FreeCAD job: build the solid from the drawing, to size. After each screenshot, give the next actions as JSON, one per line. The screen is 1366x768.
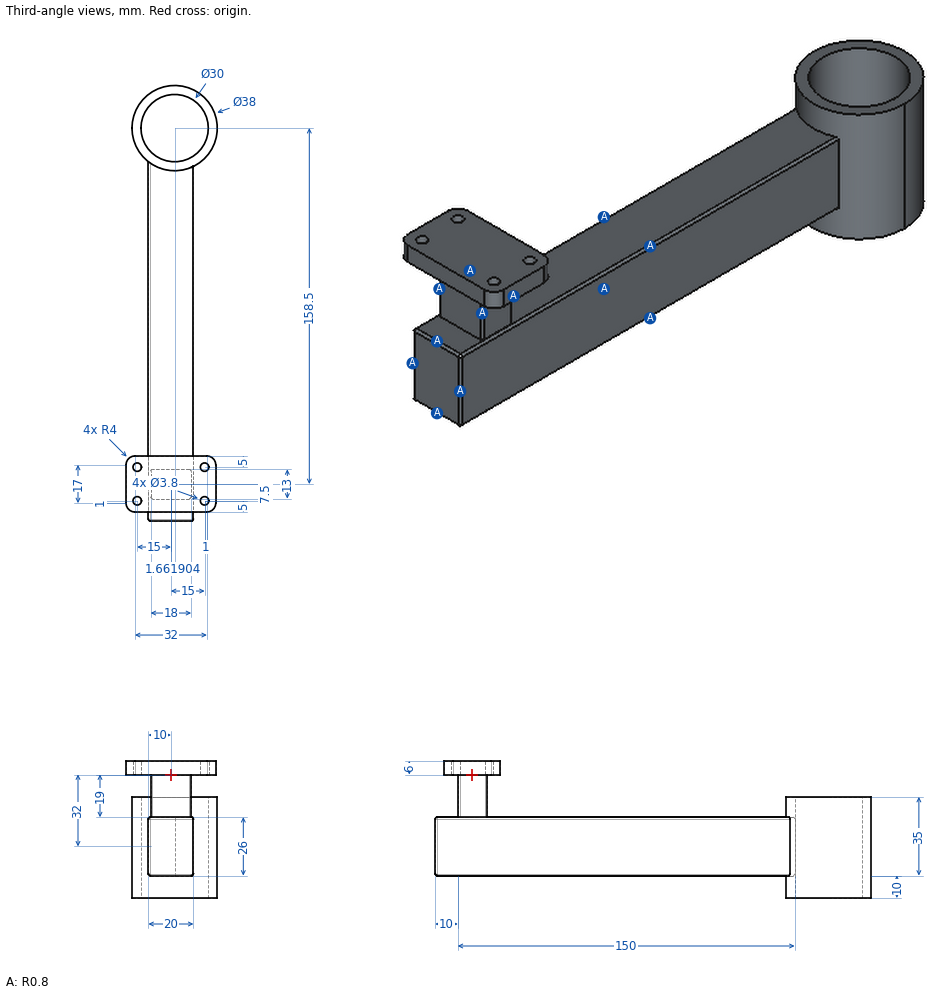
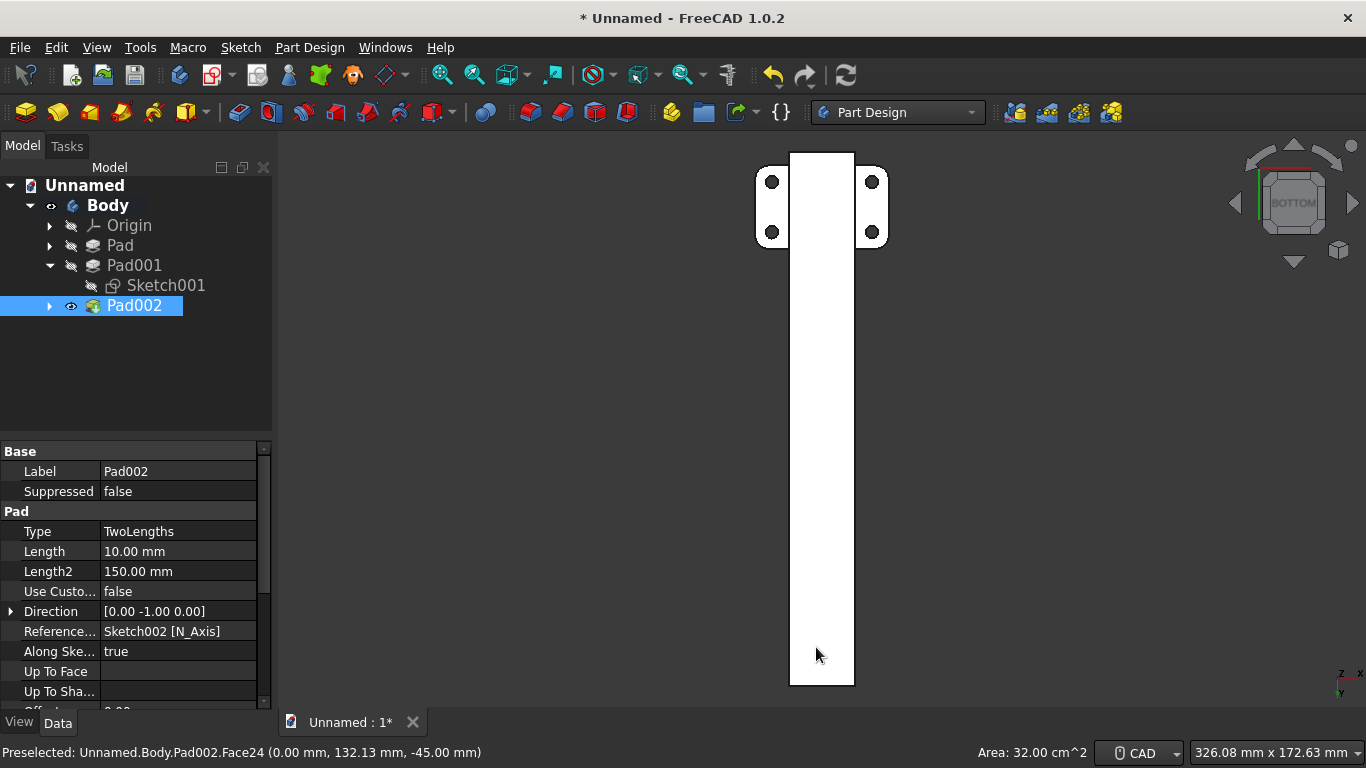
{"action": "left_click", "coordinate": [212, 76]}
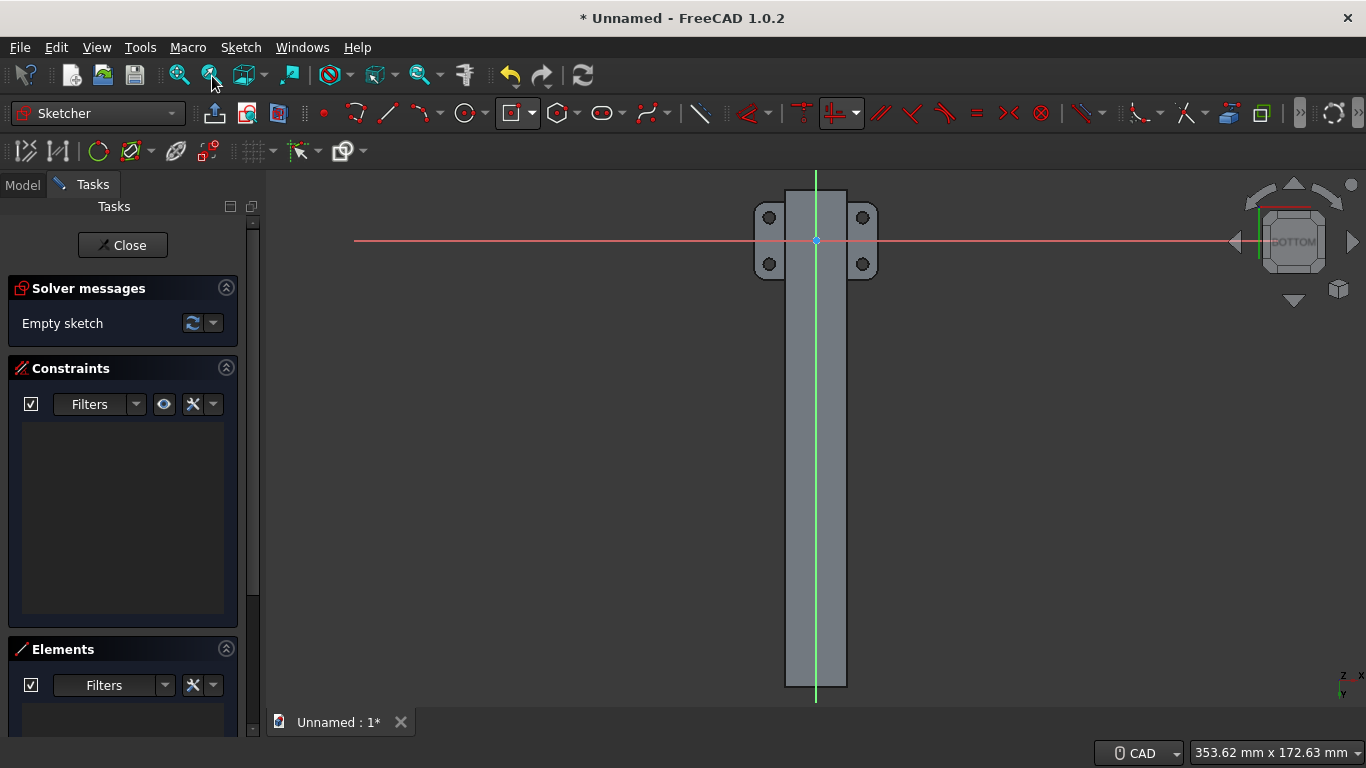
{"action": "scroll", "coordinate": [748, 438], "scroll_direction": "down", "scroll_amount": 5}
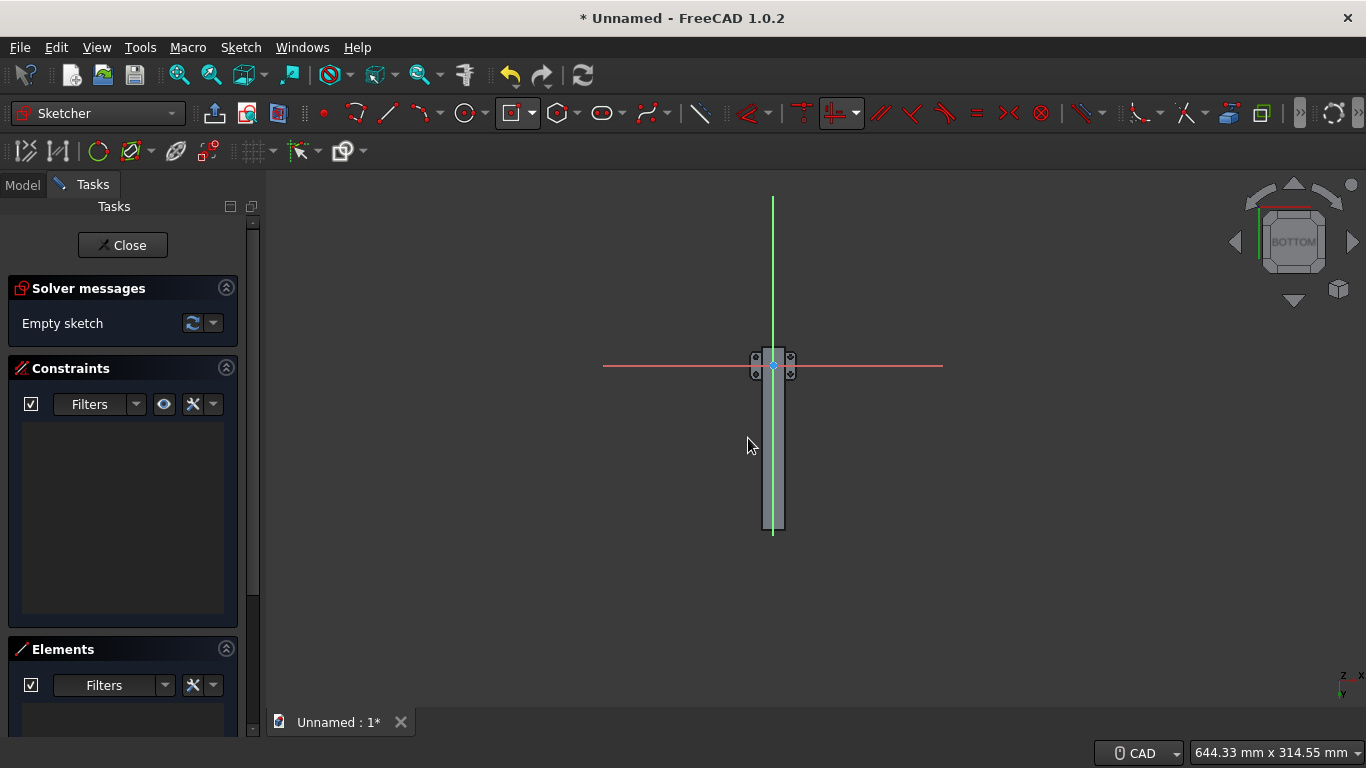
{"action": "scroll", "coordinate": [780, 564], "scroll_direction": "up", "scroll_amount": 10}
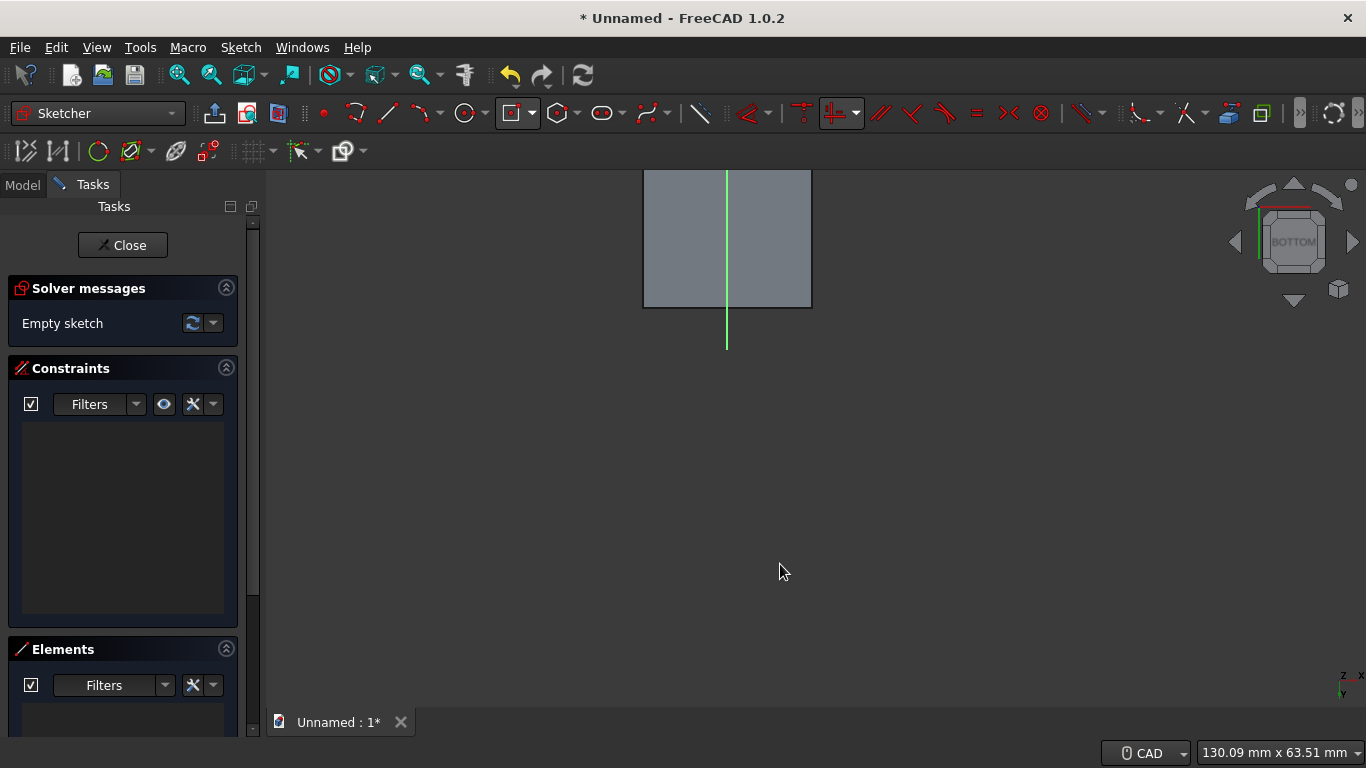
{"action": "left_click", "coordinate": [466, 114]}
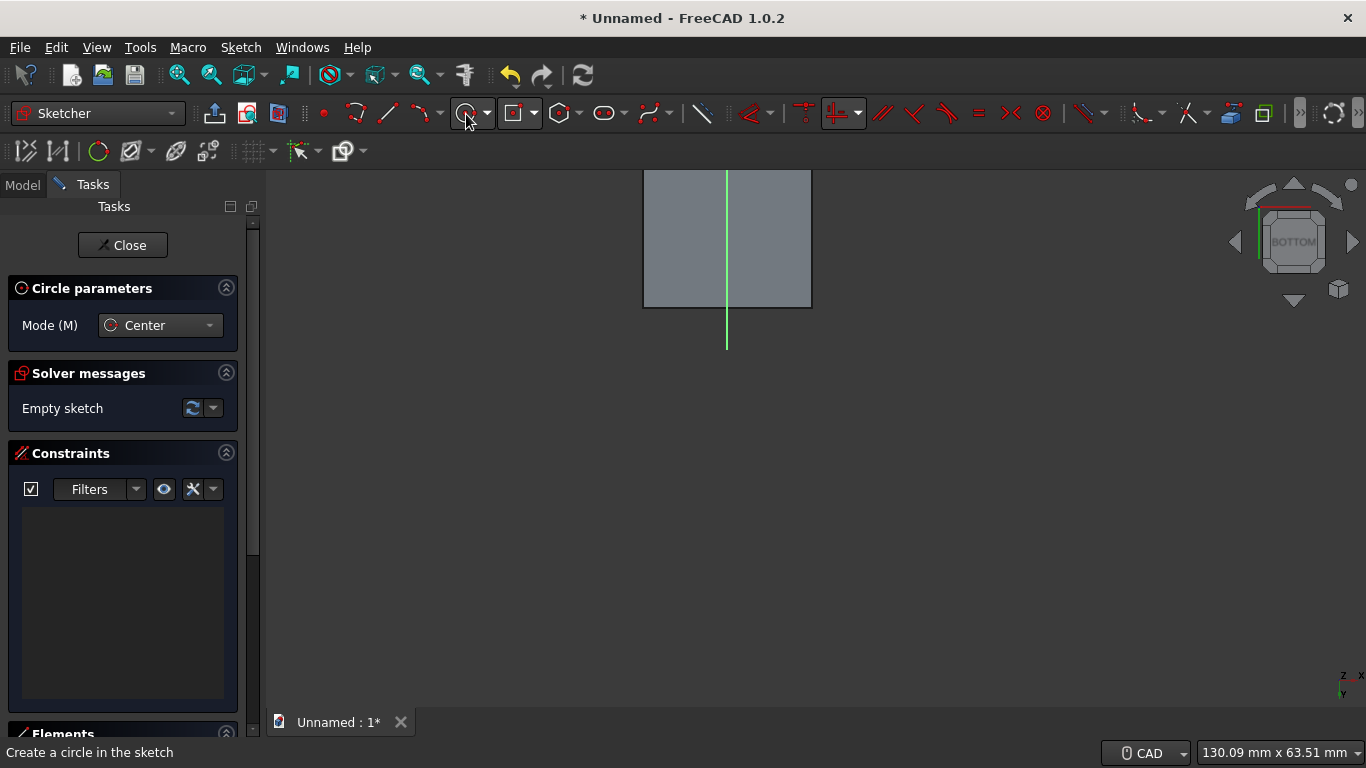
{"action": "left_click", "coordinate": [742, 435]}
{"action": "mouse_move", "coordinate": [855, 322]}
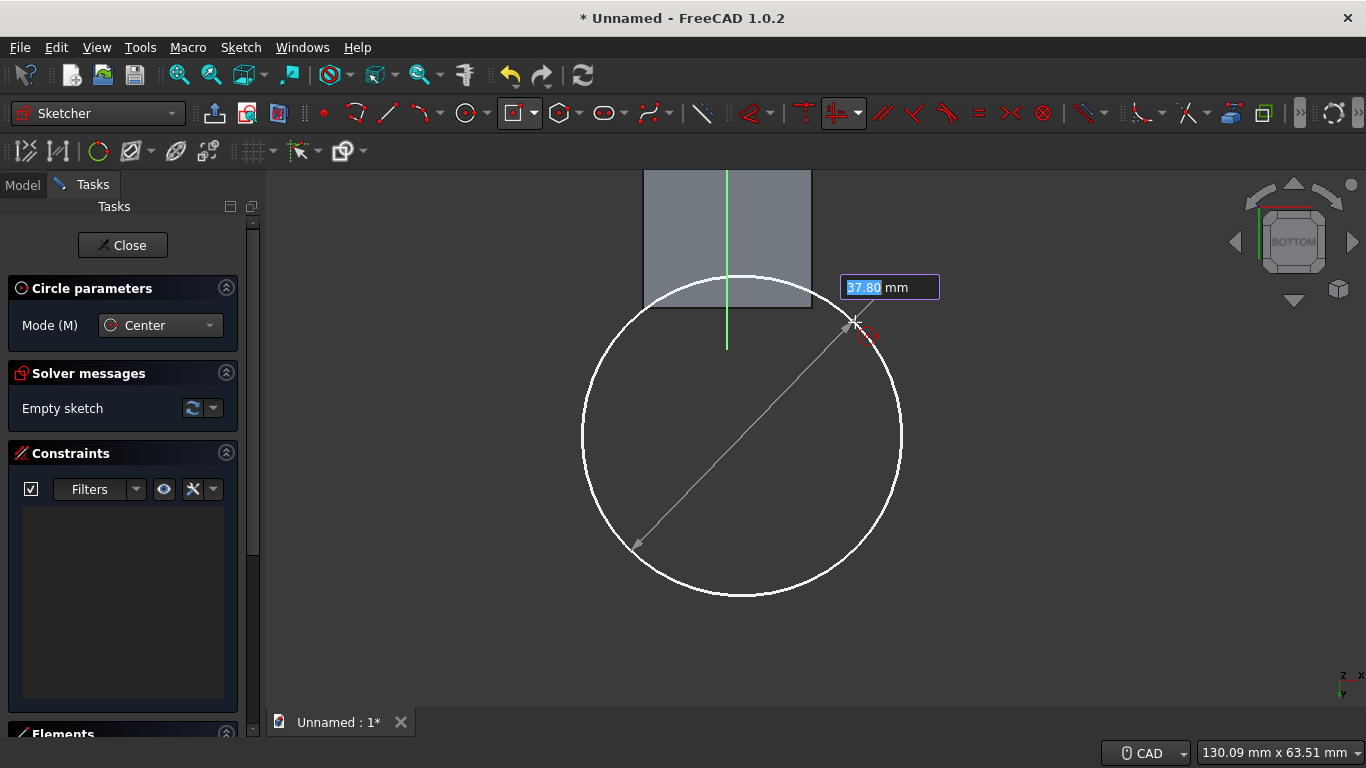
{"action": "type", "text": "38"}
{"action": "key", "text": "Return"}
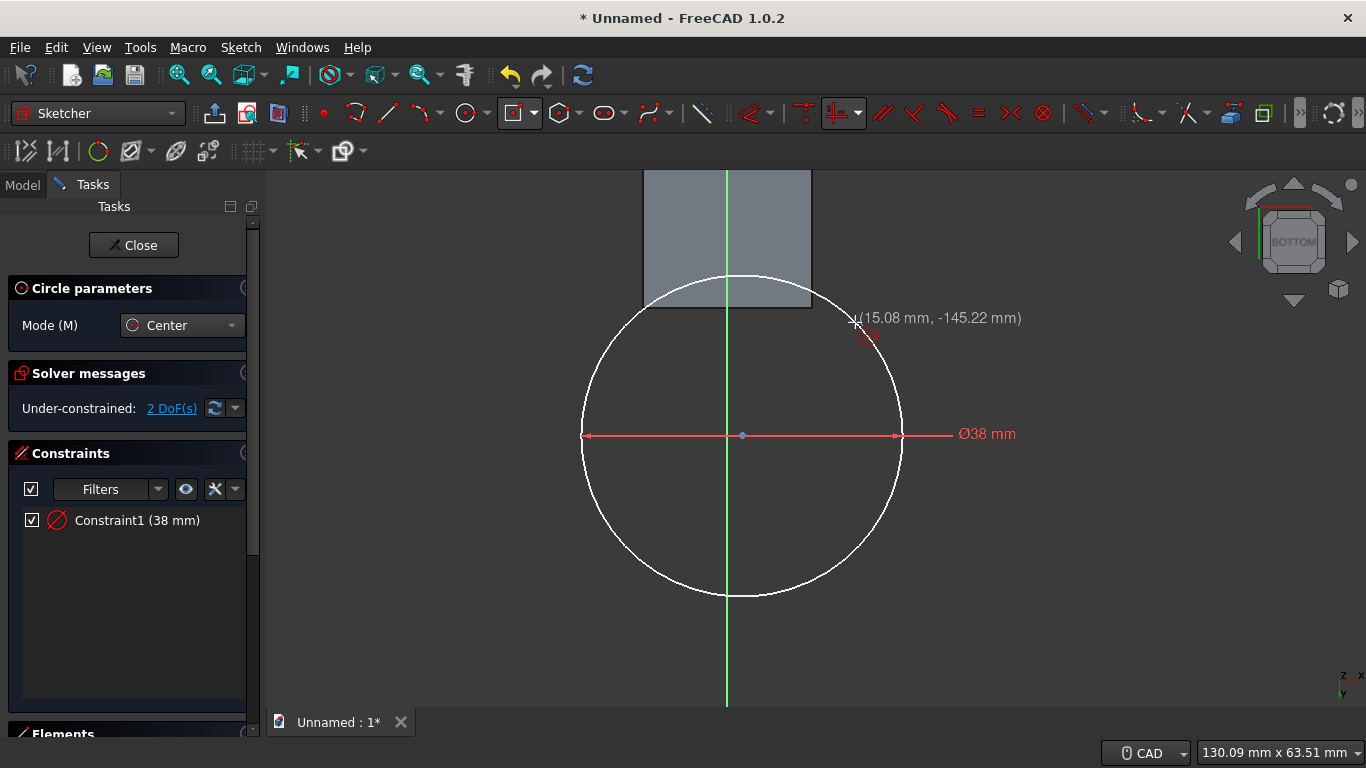
{"action": "left_click", "coordinate": [742, 436]}
{"action": "mouse_move", "coordinate": [831, 346]}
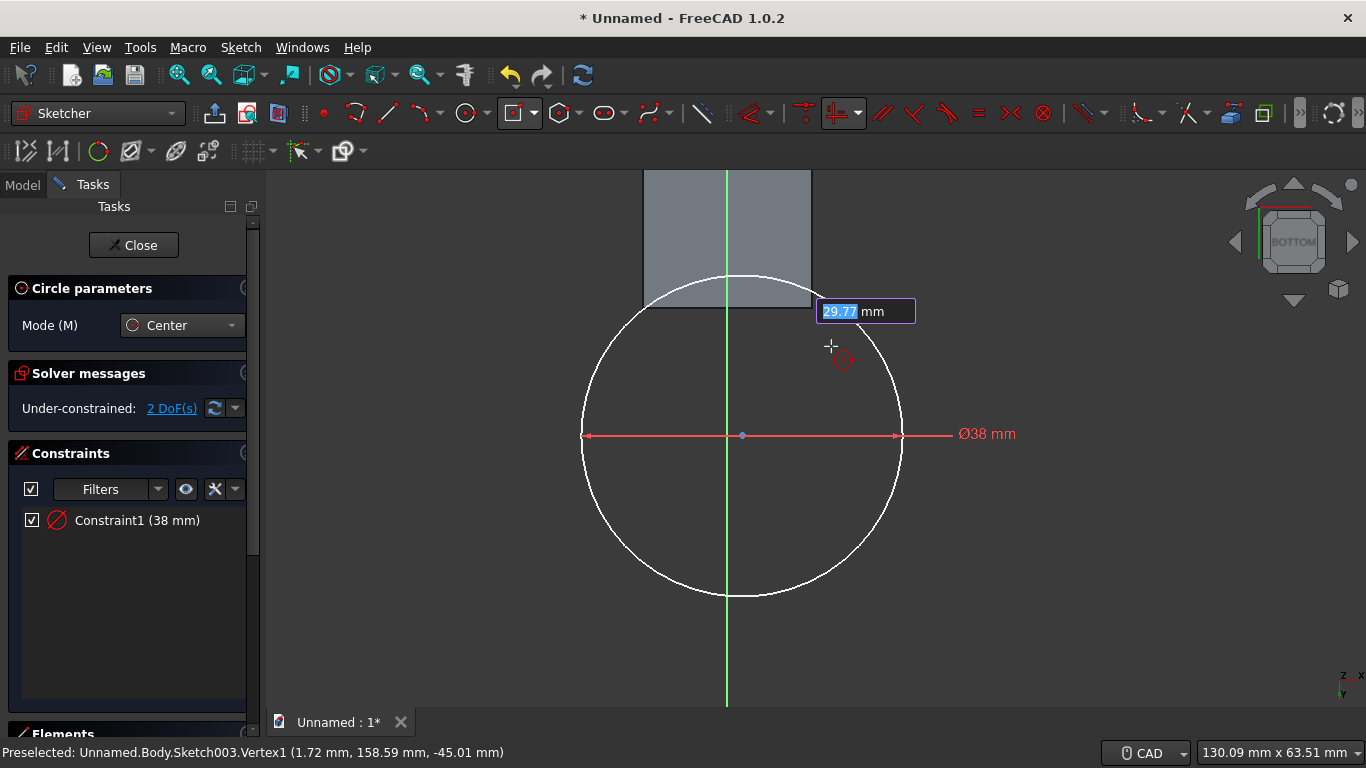
{"action": "type", "text": "30"}
{"action": "key", "text": "Return"}
{"action": "key", "text": "Escape"}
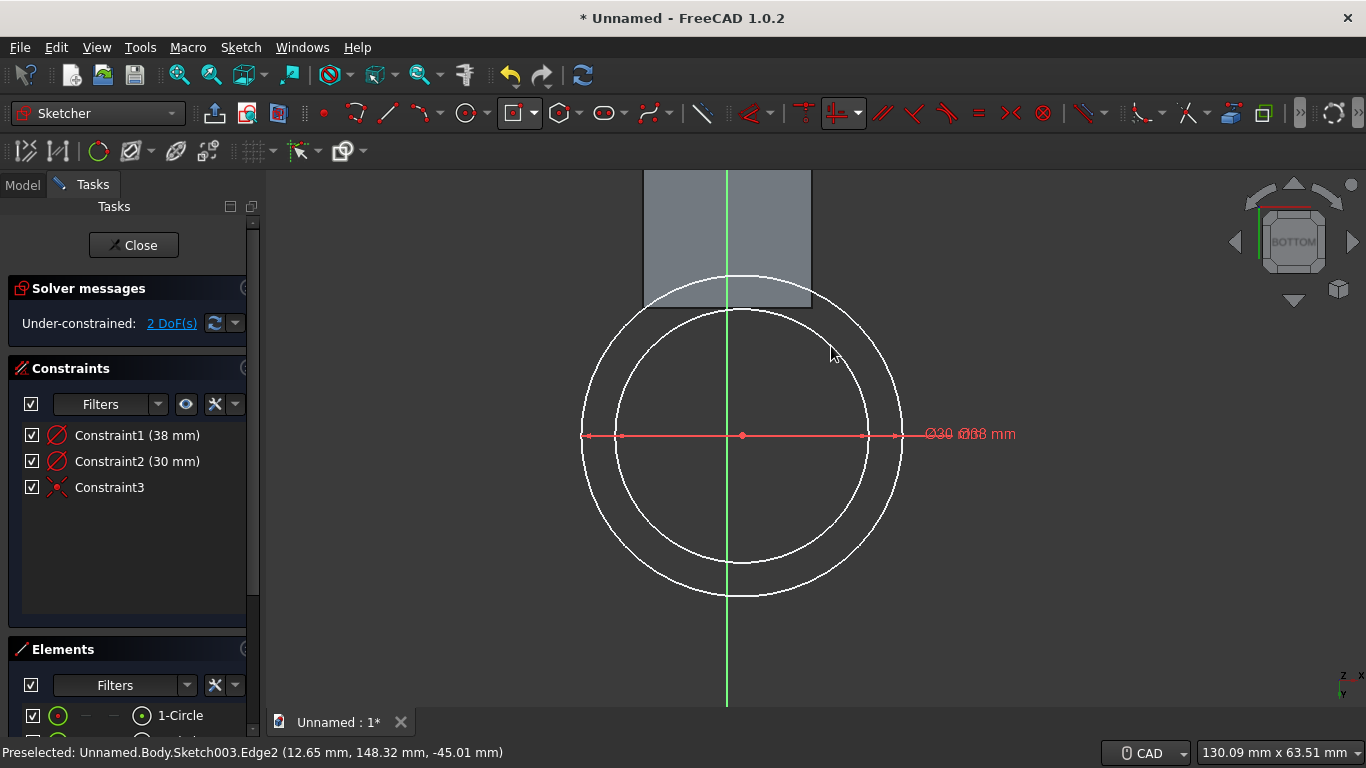
{"action": "left_click", "coordinate": [750, 114]}